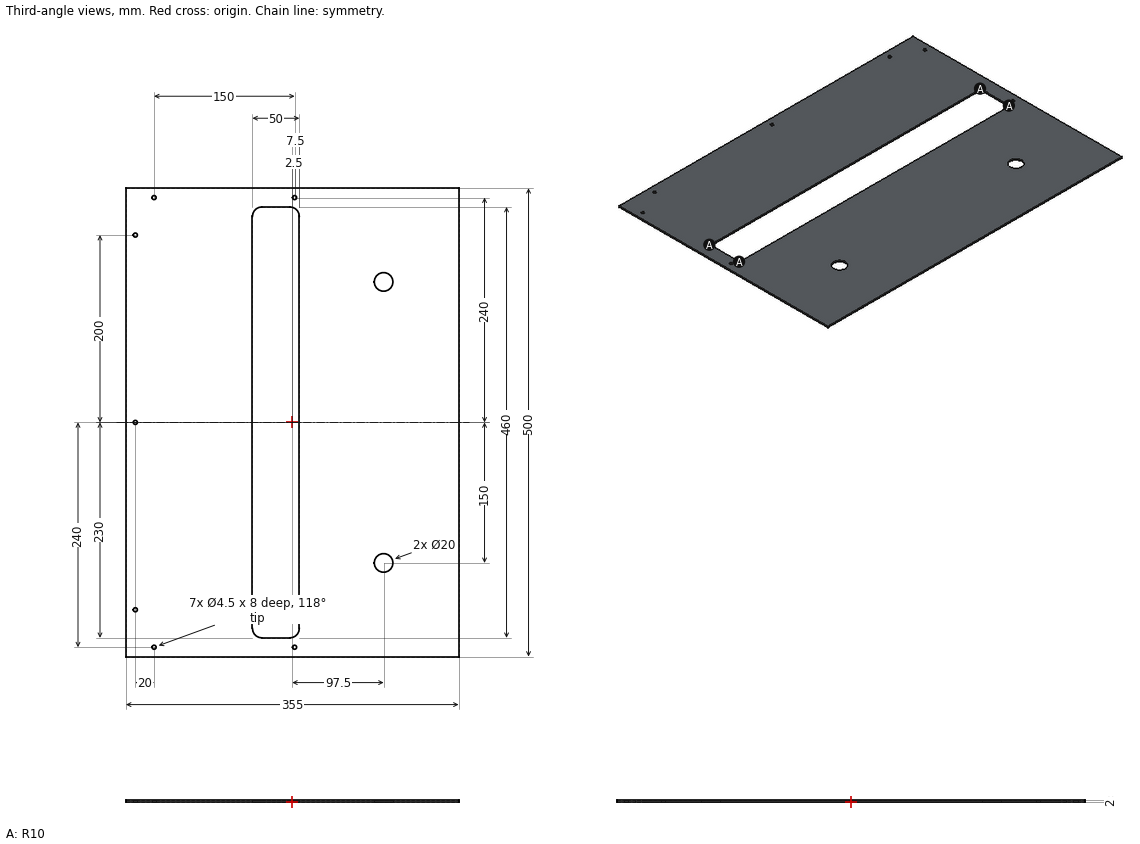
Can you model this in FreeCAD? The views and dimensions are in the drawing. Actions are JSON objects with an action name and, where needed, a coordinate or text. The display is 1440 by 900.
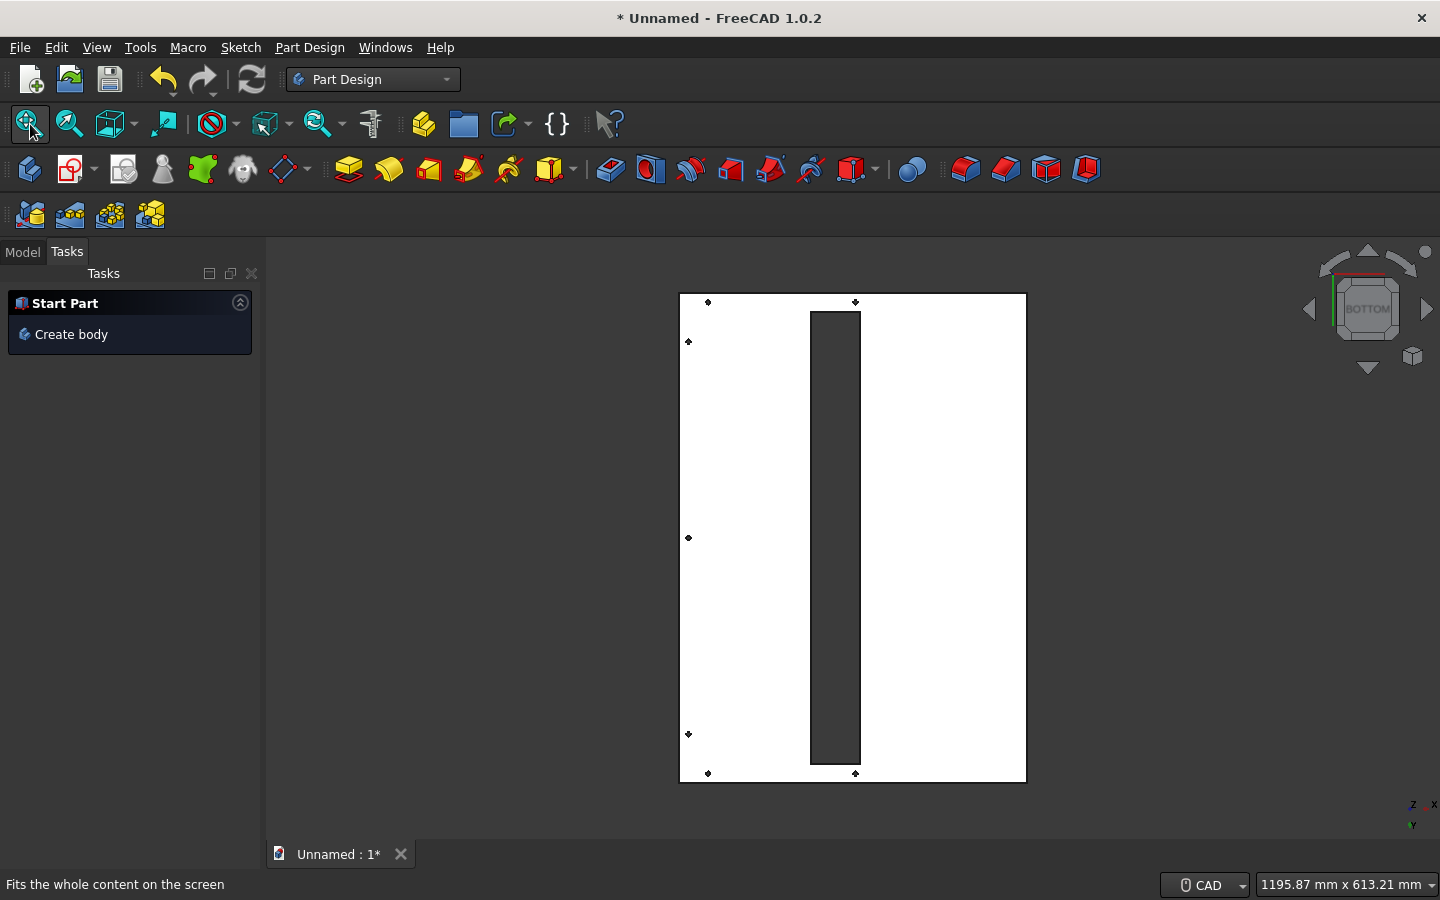
{"action": "key", "text": "0"}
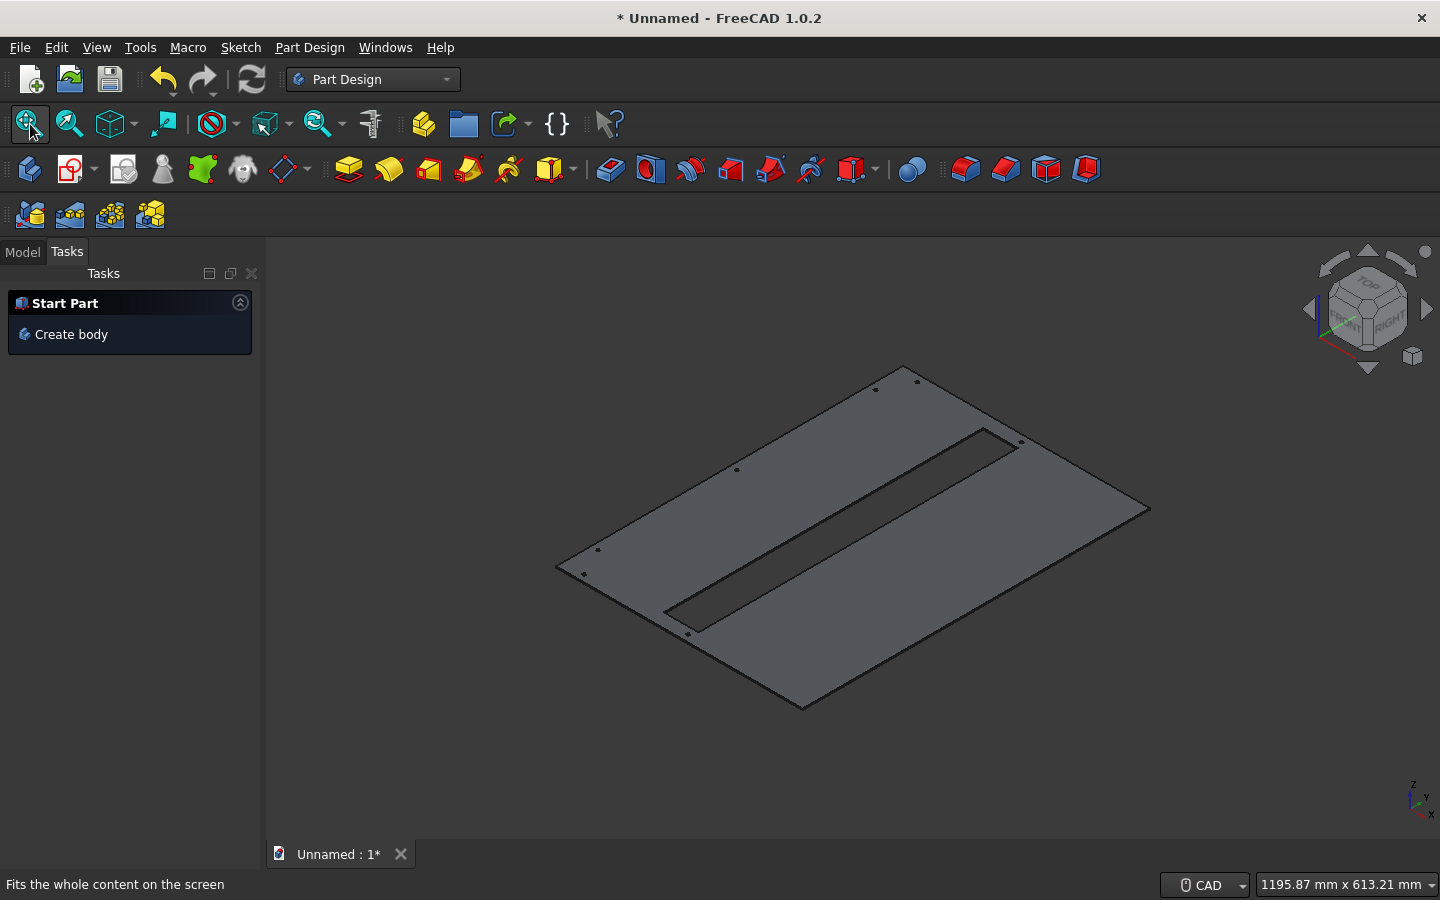
{"action": "scroll", "coordinate": [983, 428], "scroll_direction": "up", "scroll_amount": 15}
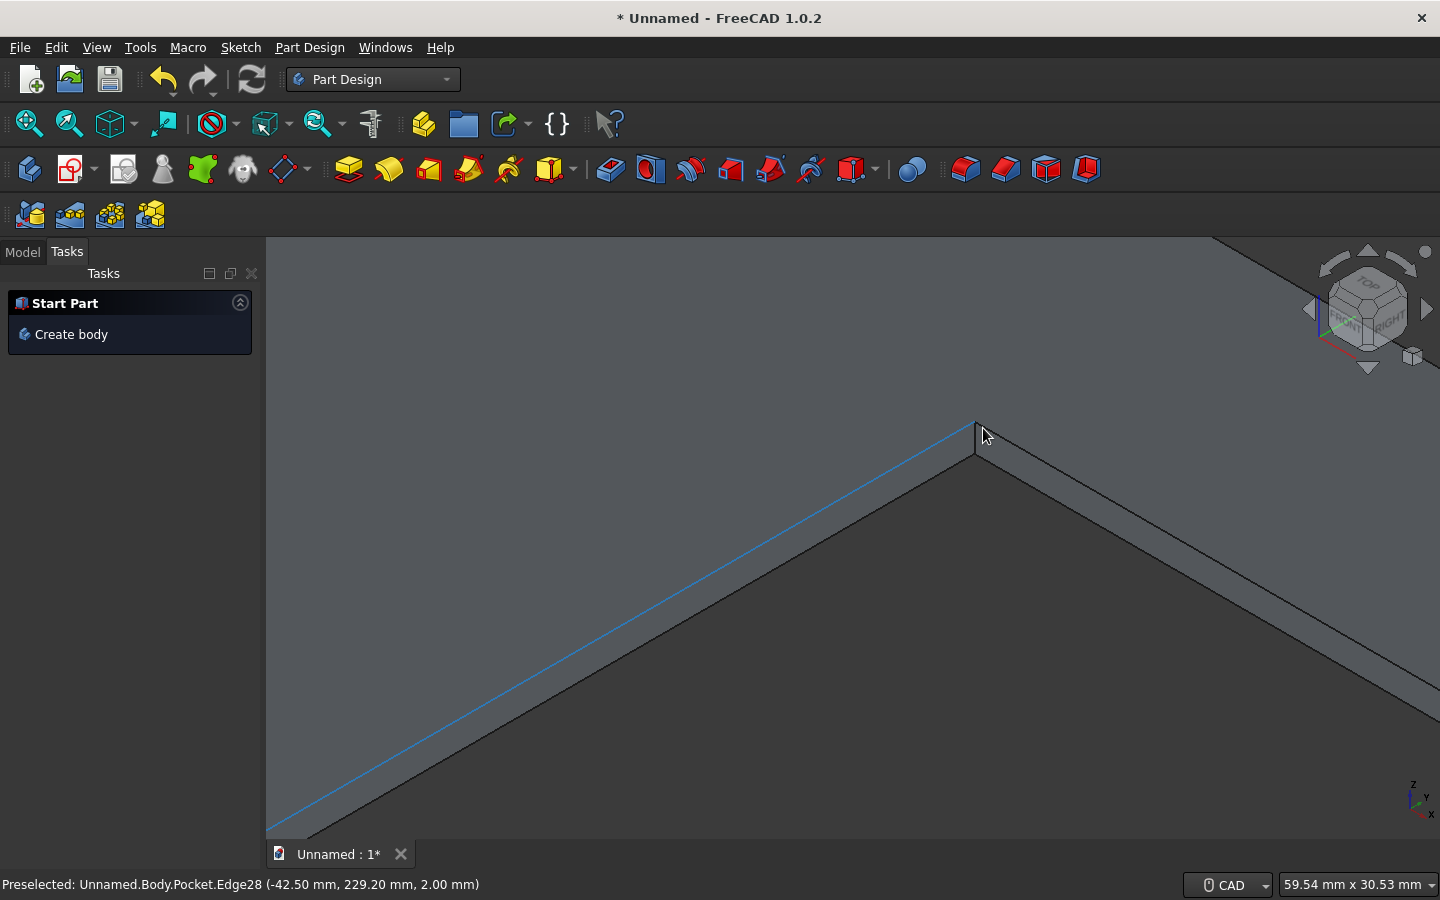
{"action": "left_click", "coordinate": [30, 124]}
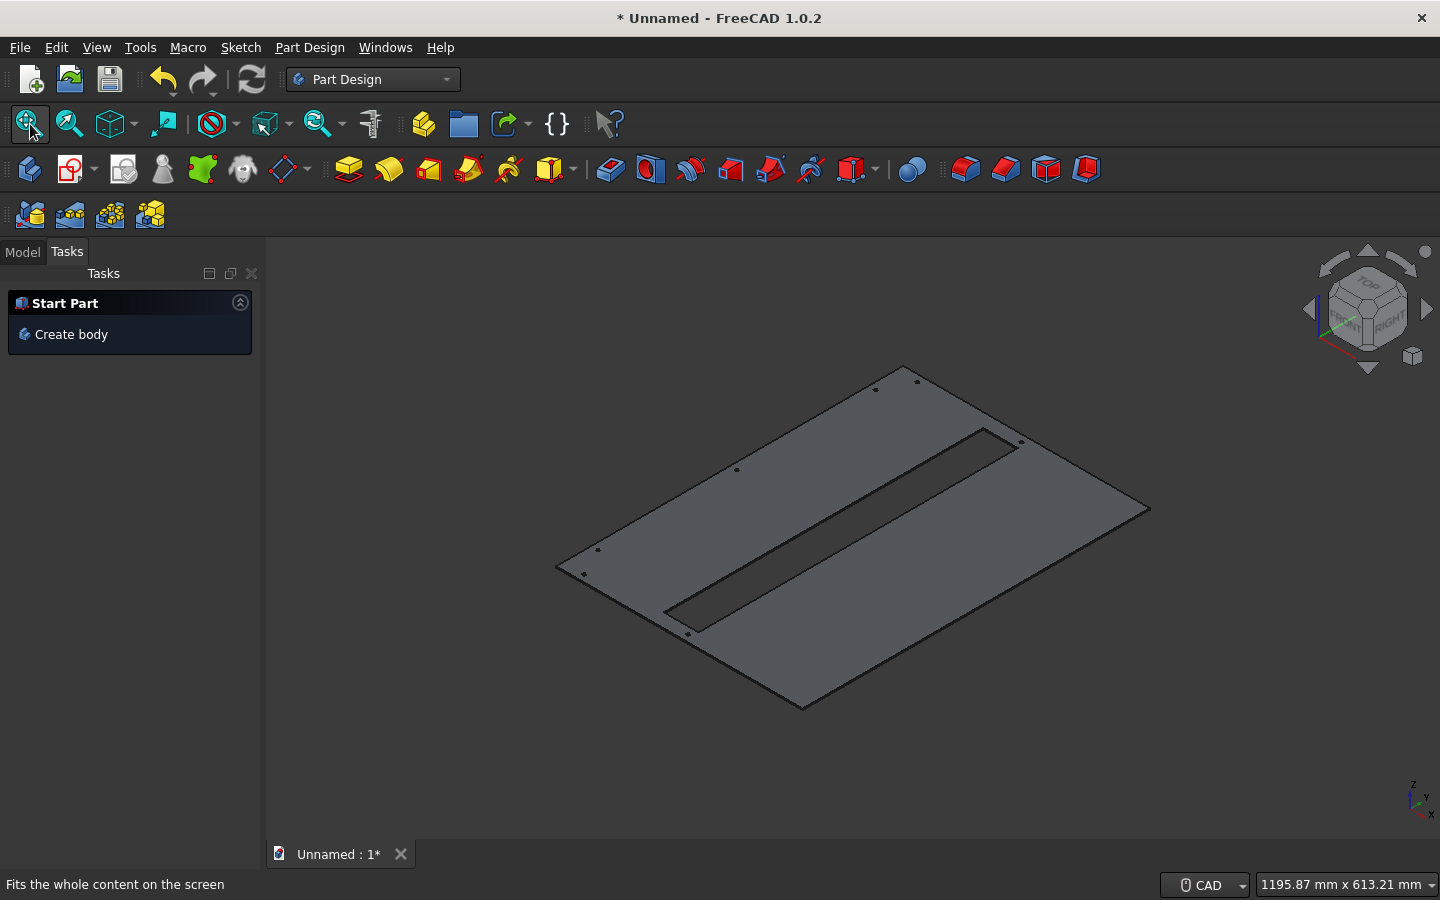
{"action": "key", "text": "2"}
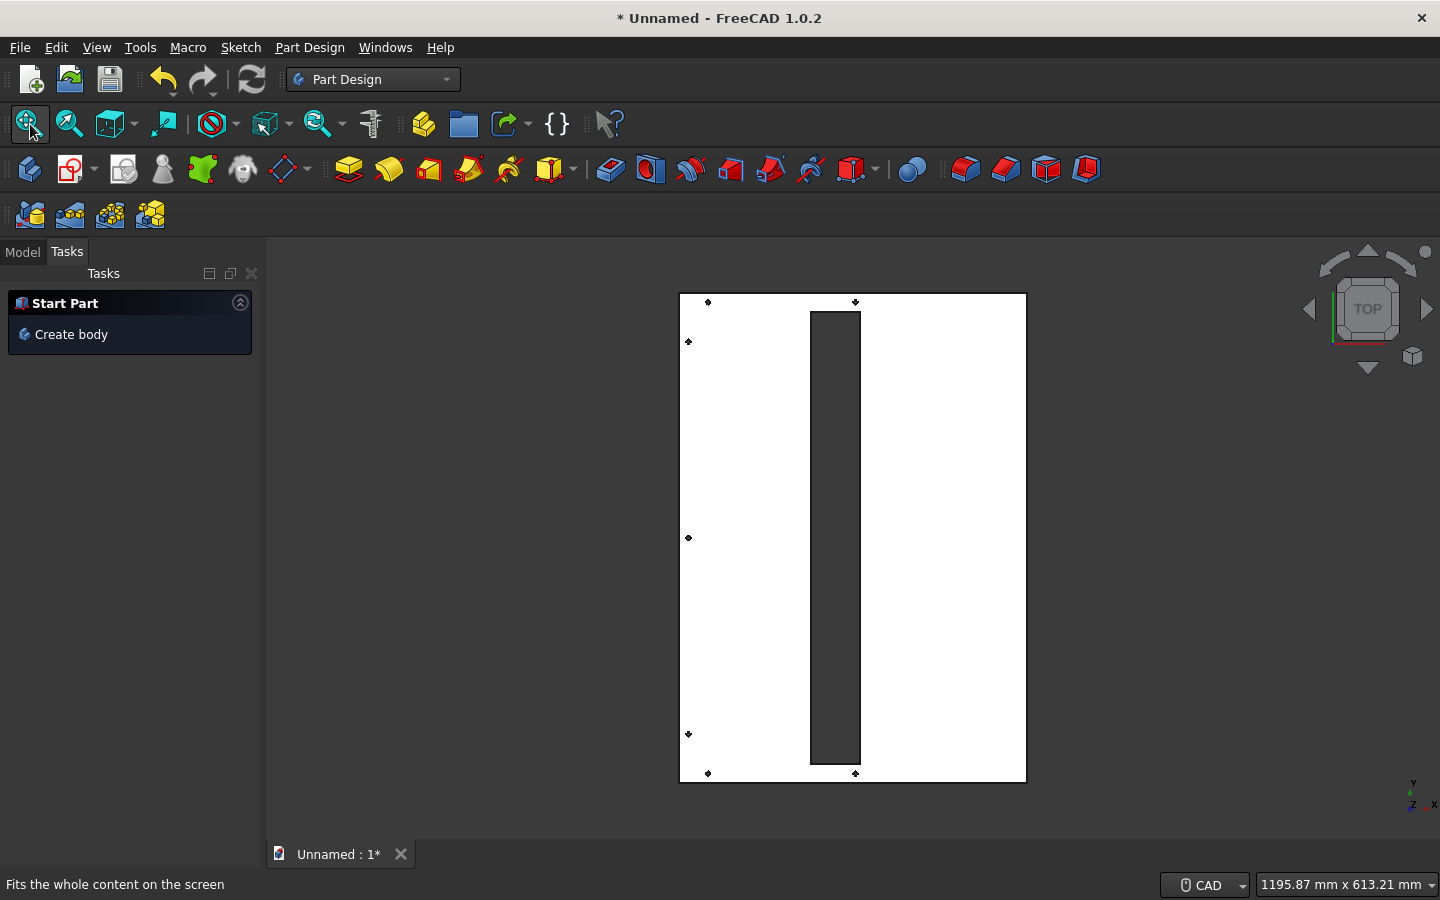
{"action": "scroll", "coordinate": [811, 311], "scroll_direction": "up", "scroll_amount": 15}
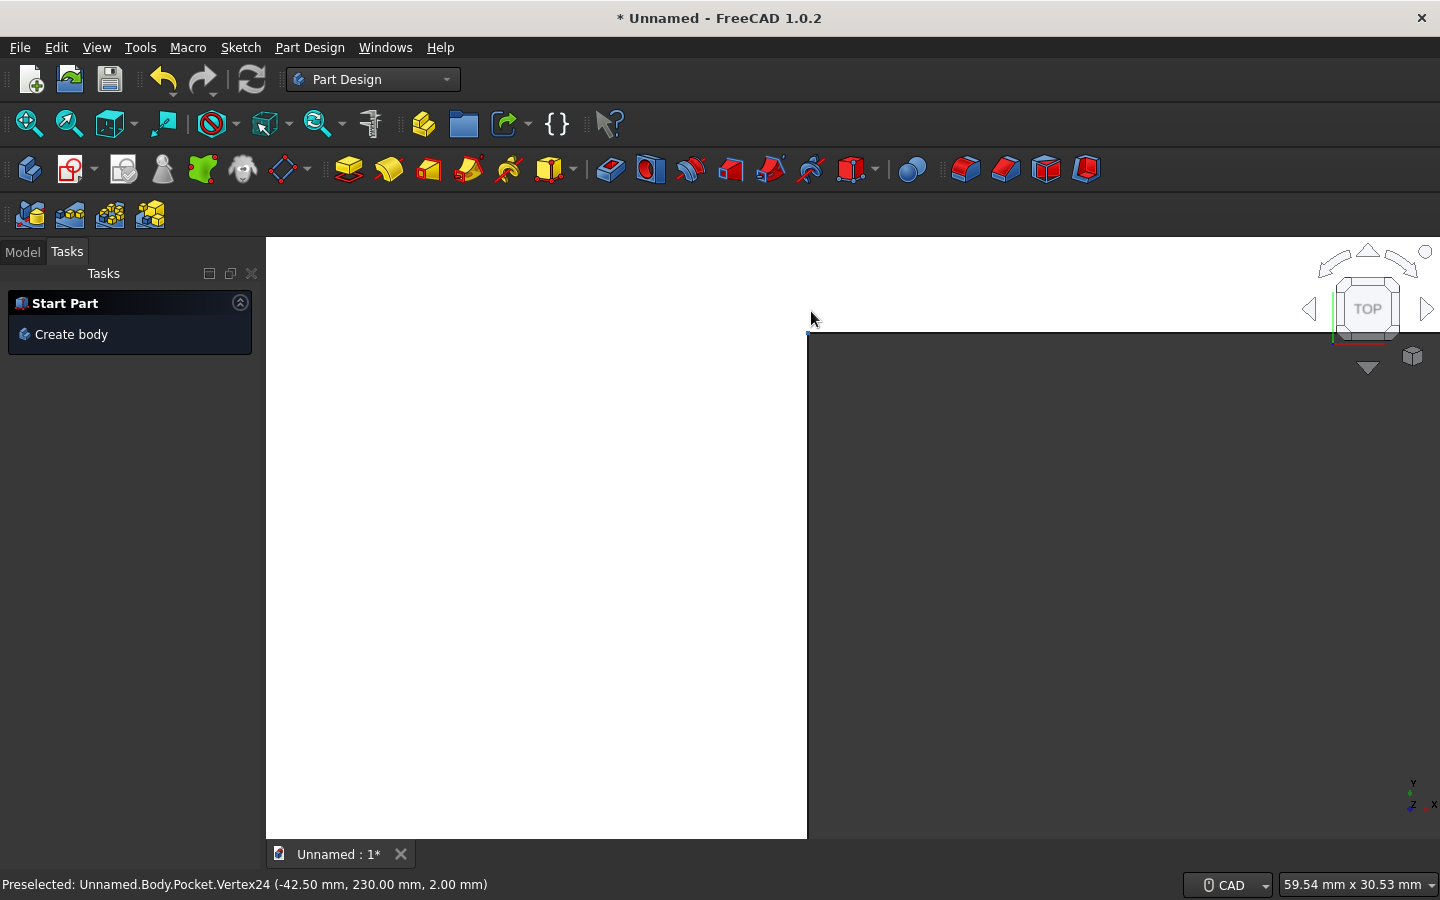
{"action": "left_click", "coordinate": [30, 124]}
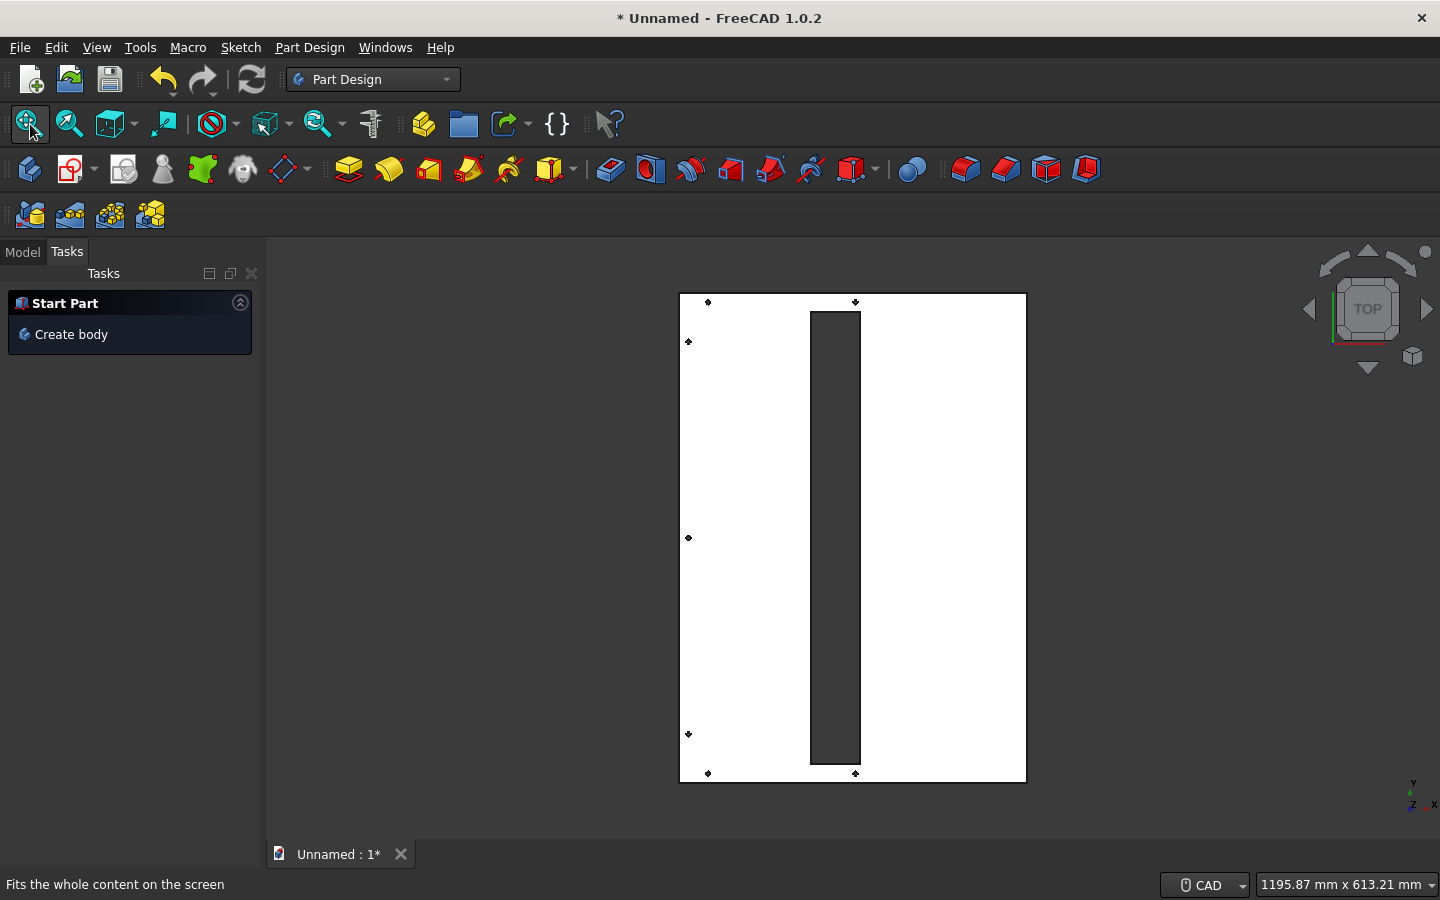
{"action": "key", "text": "1"}